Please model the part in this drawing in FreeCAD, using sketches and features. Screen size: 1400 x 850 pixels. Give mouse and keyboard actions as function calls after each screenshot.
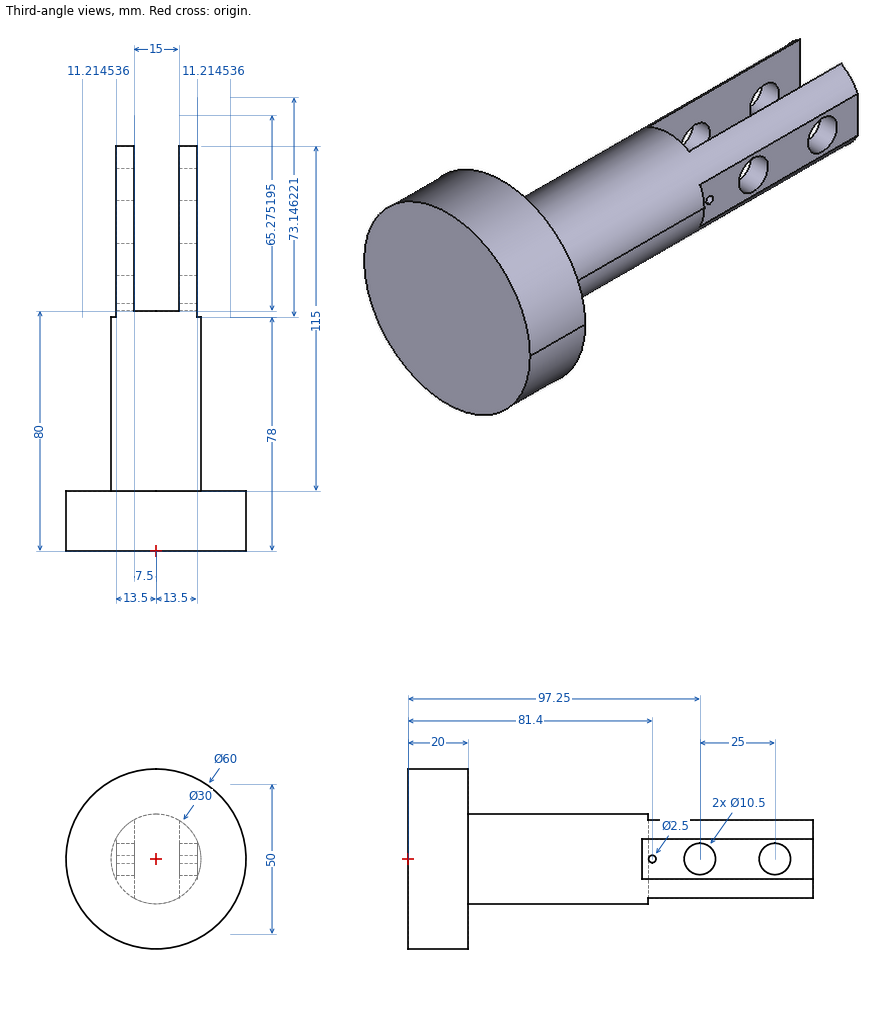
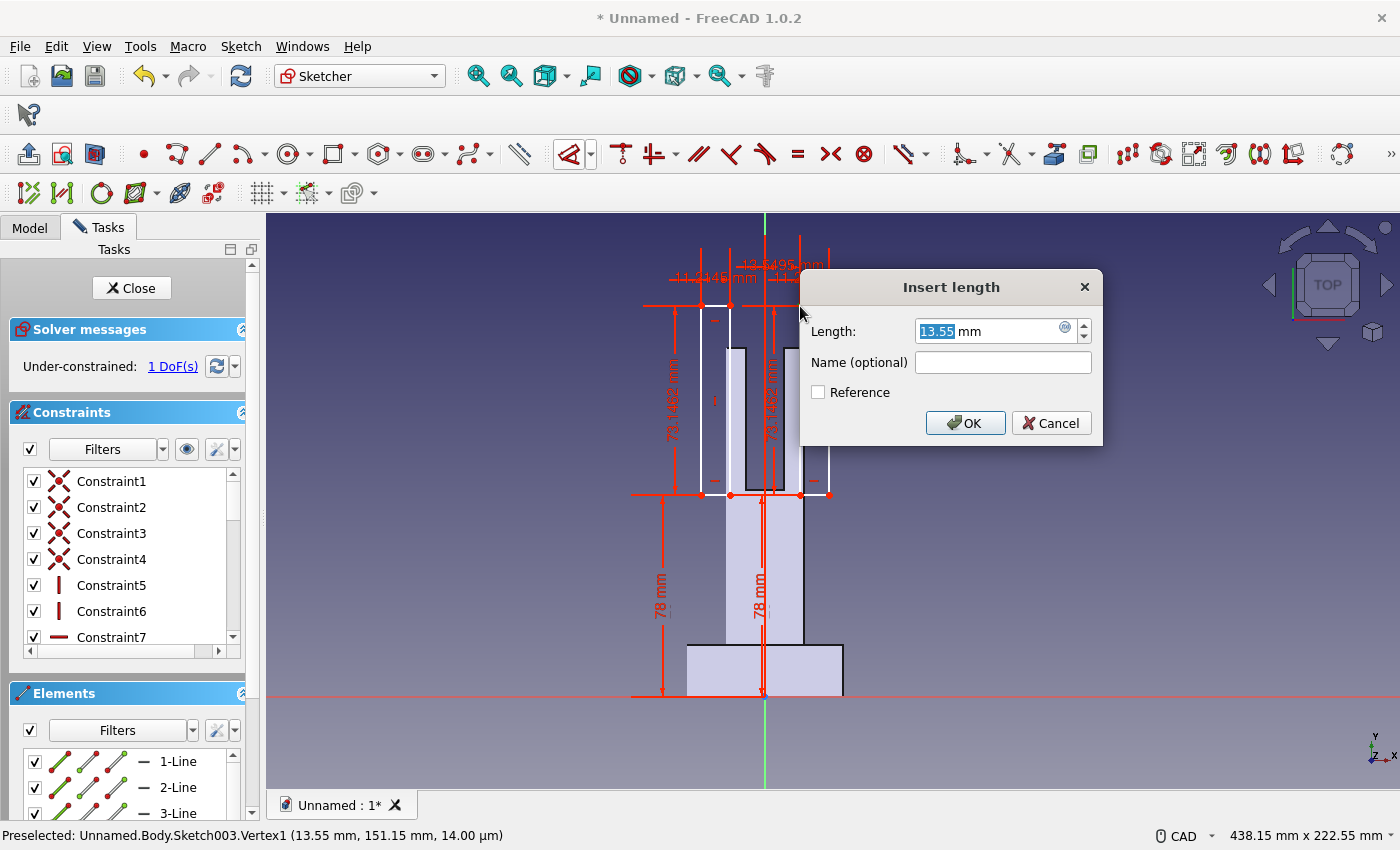
text(13.5)
key(Return)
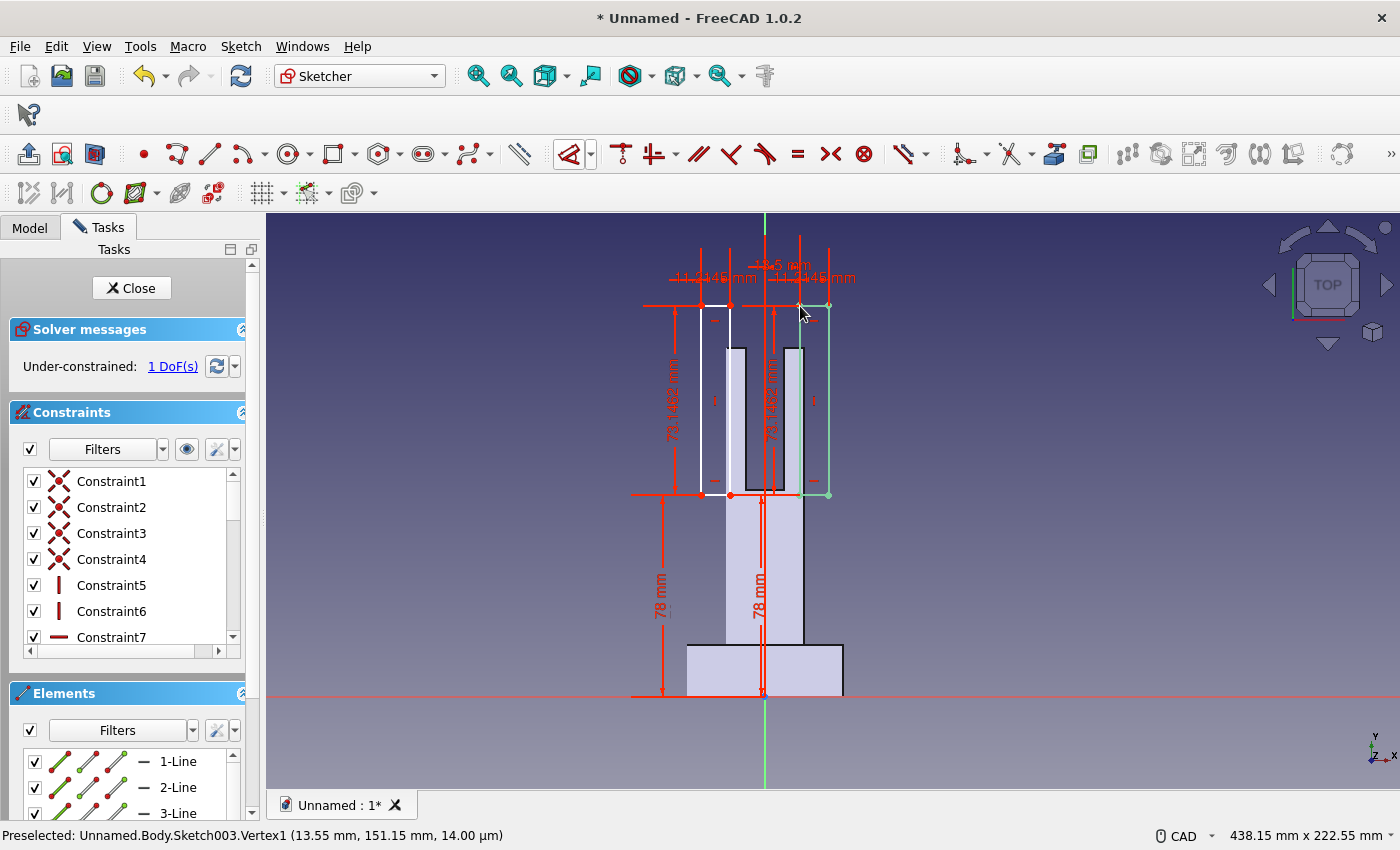
click(730, 495)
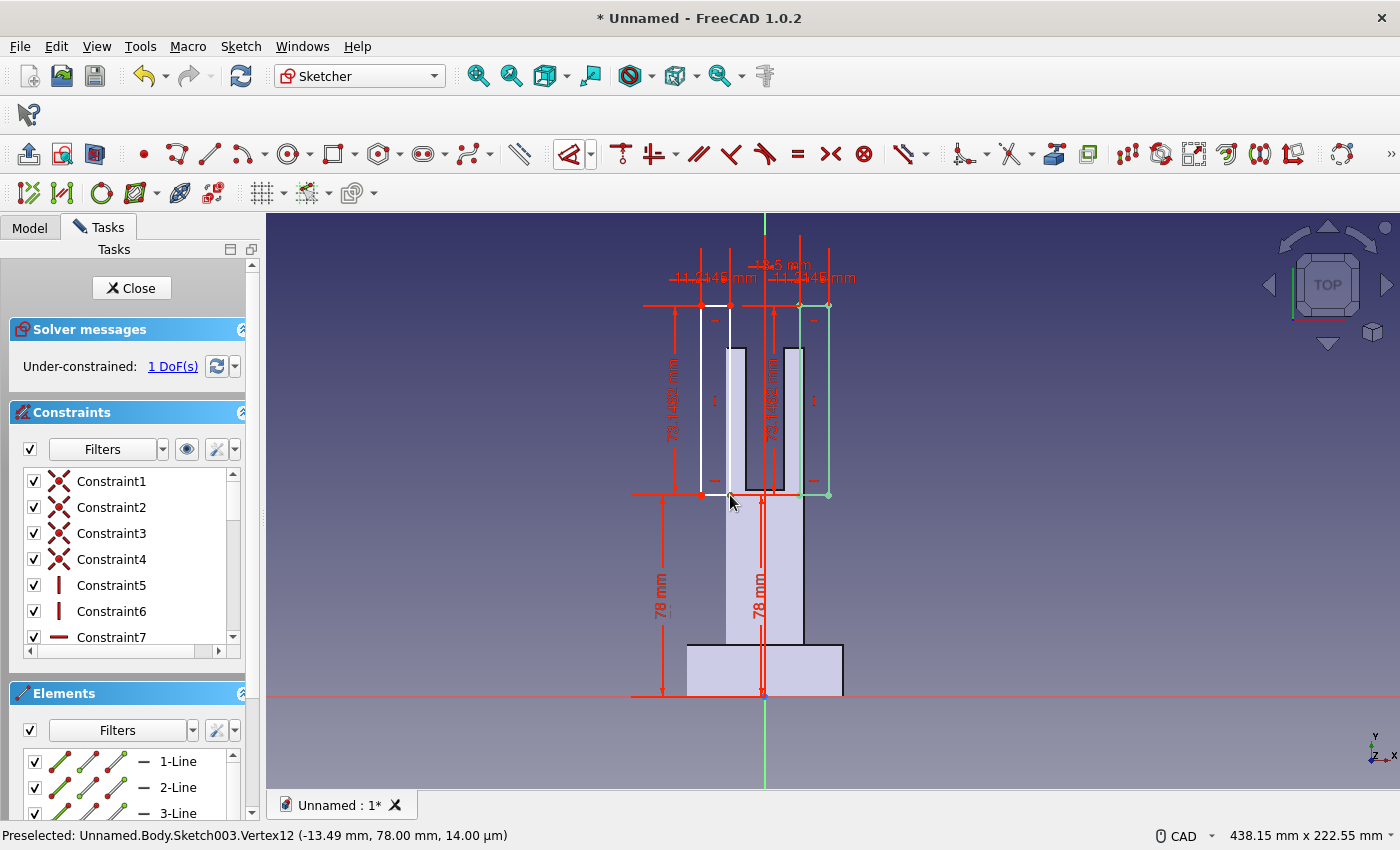
click(590, 154)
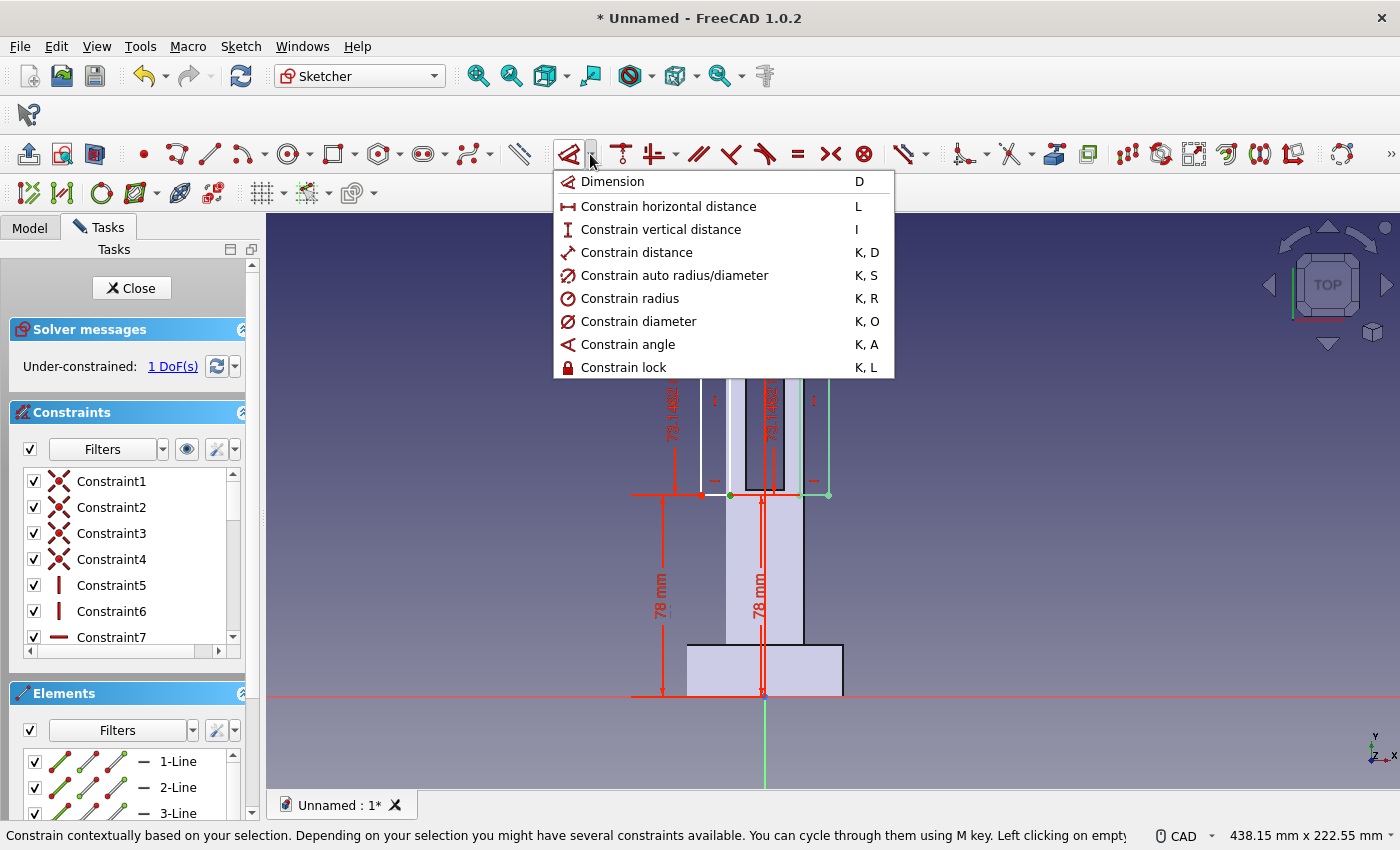
click(724, 206)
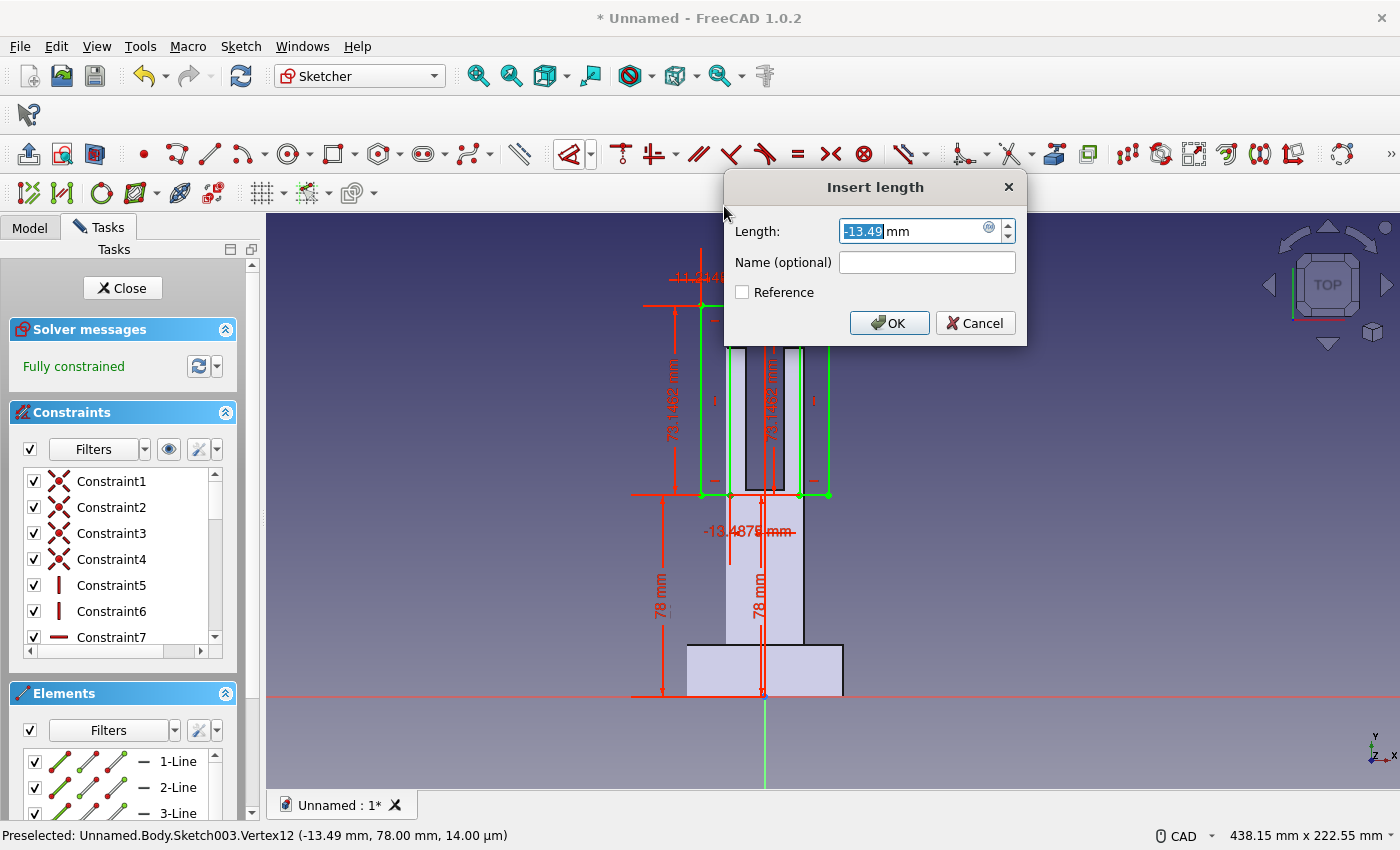
text(-13.5)
key(Return)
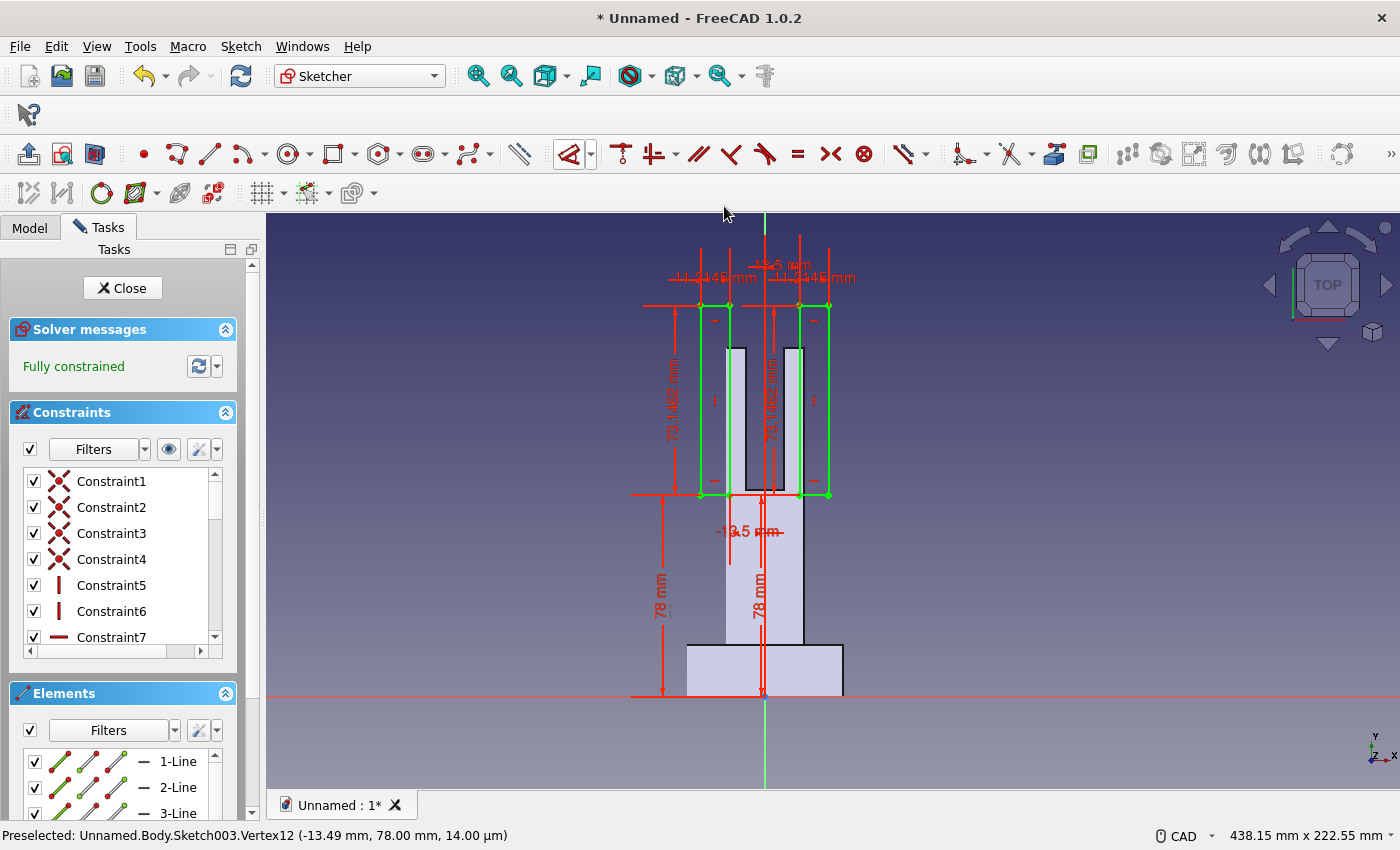
click(123, 288)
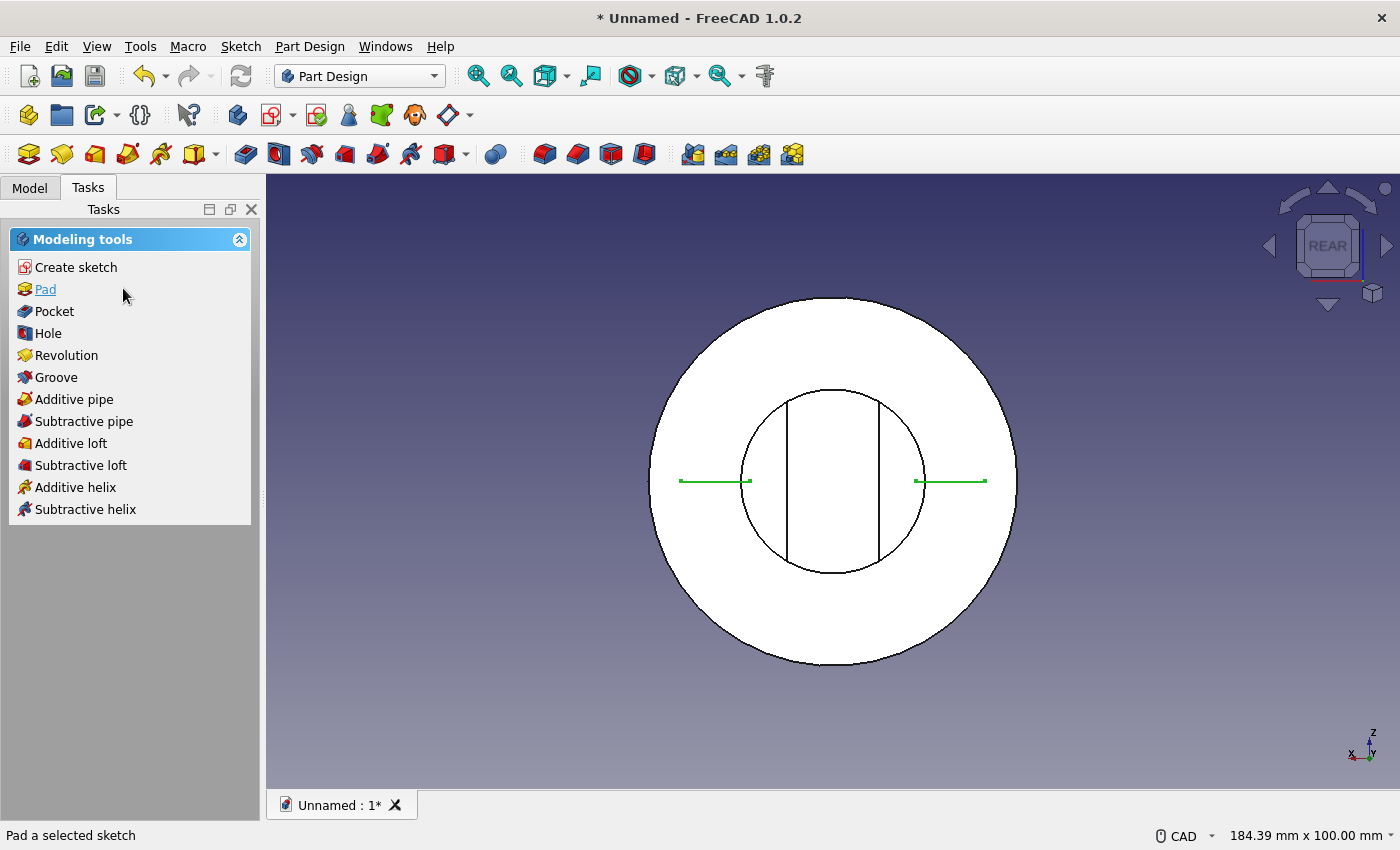
click(246, 154)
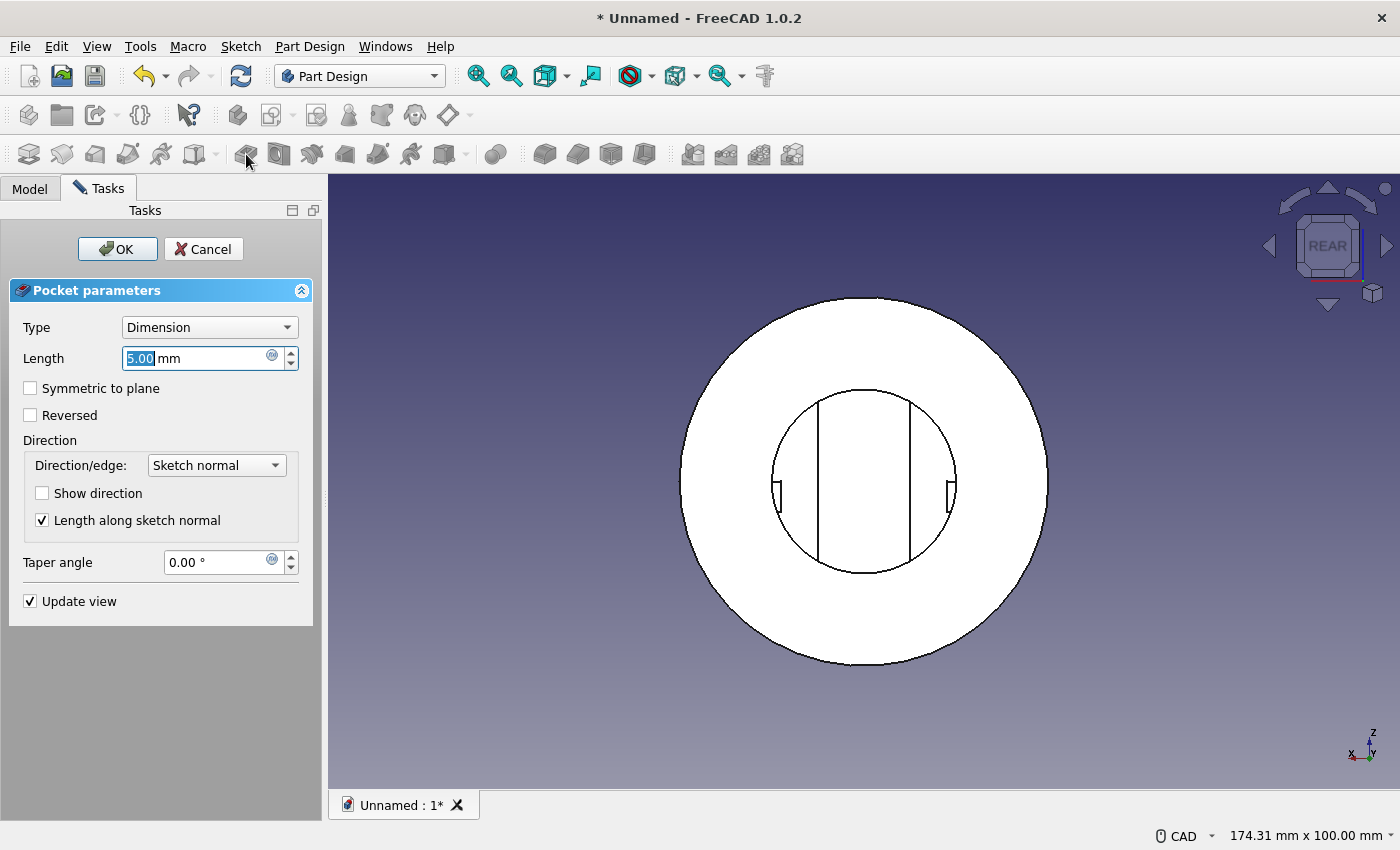
text(50)
key(Tab)